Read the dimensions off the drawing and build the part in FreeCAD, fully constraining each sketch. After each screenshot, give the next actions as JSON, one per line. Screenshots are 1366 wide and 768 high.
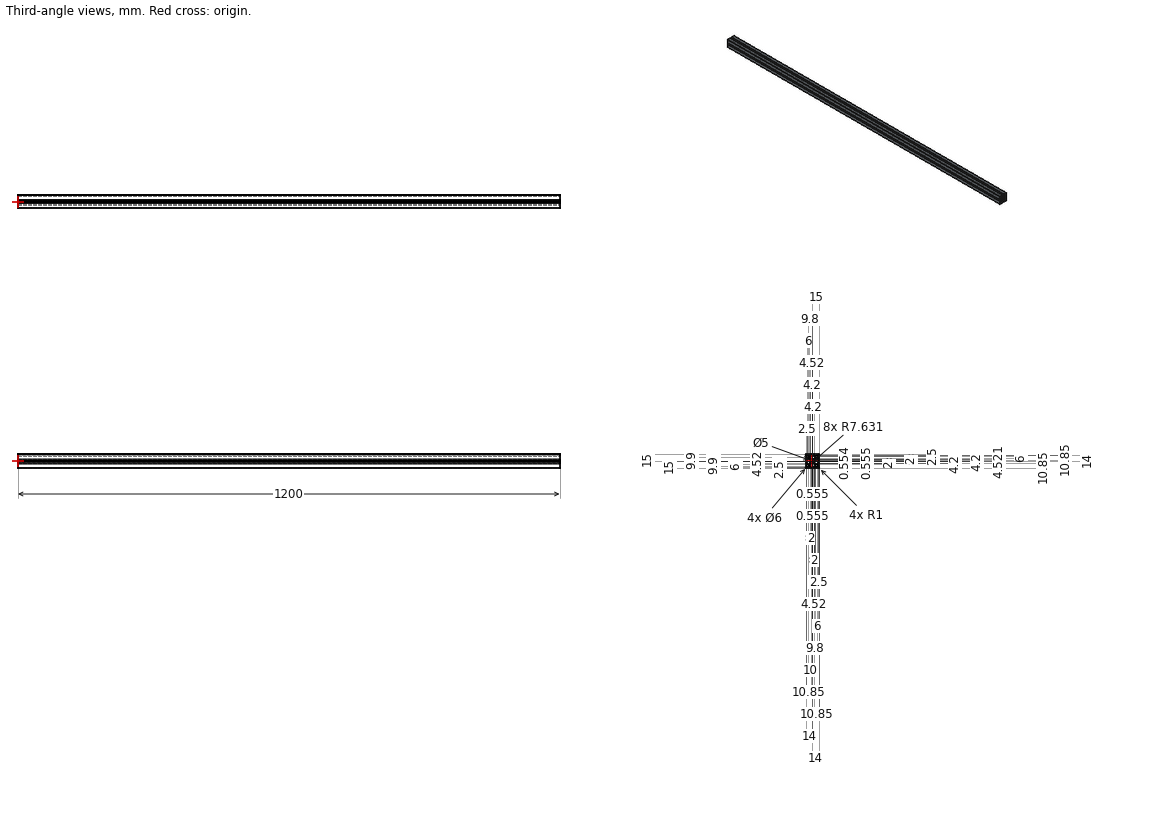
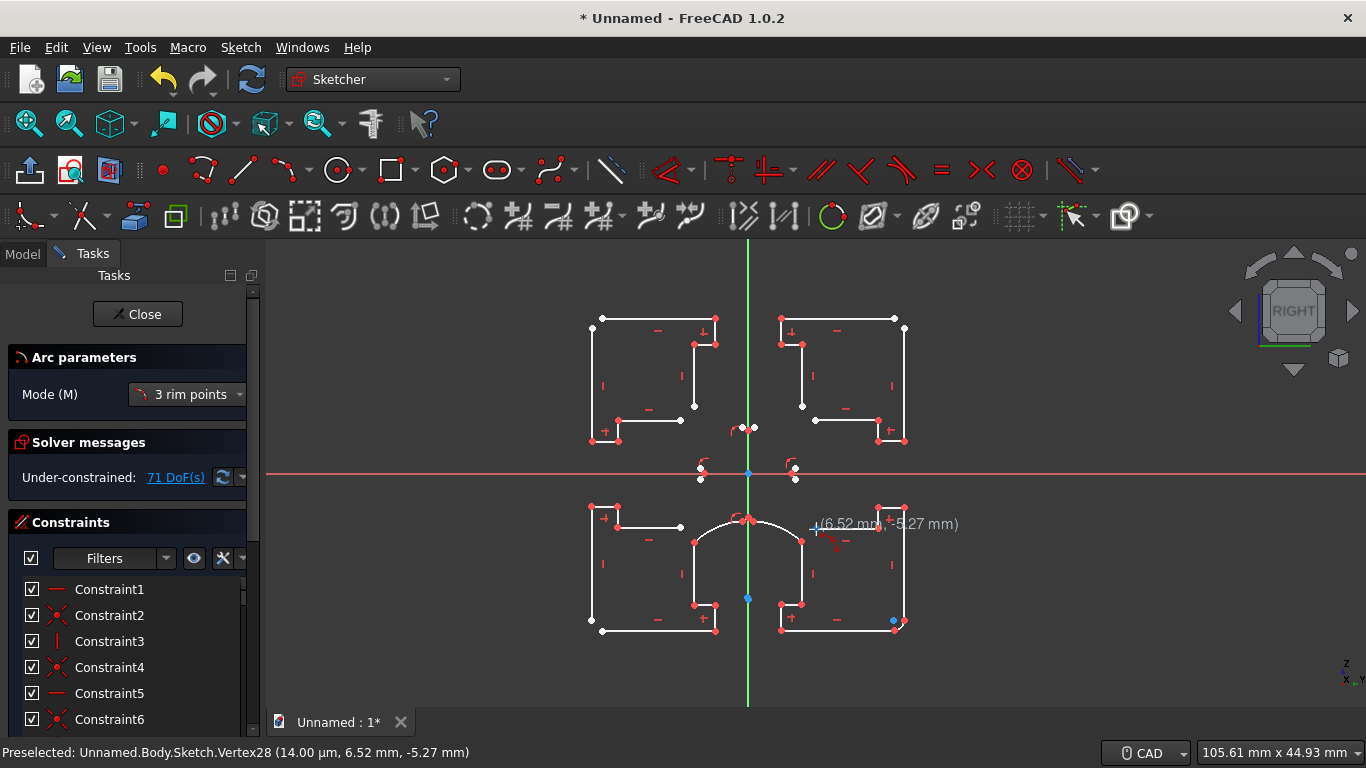
{"action": "scroll", "coordinate": [795, 480], "scroll_direction": "up", "scroll_amount": 8}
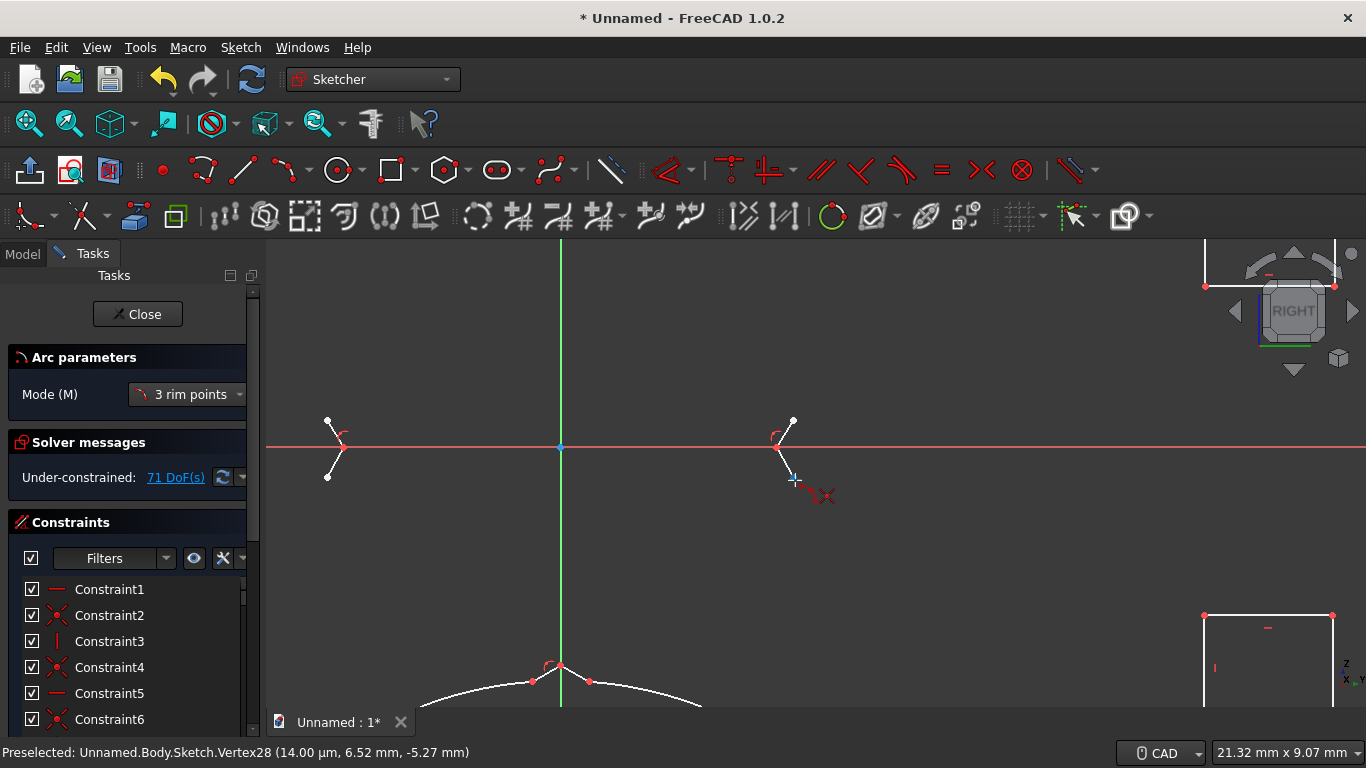
{"action": "left_click", "coordinate": [793, 477]}
{"action": "left_click", "coordinate": [825, 603]}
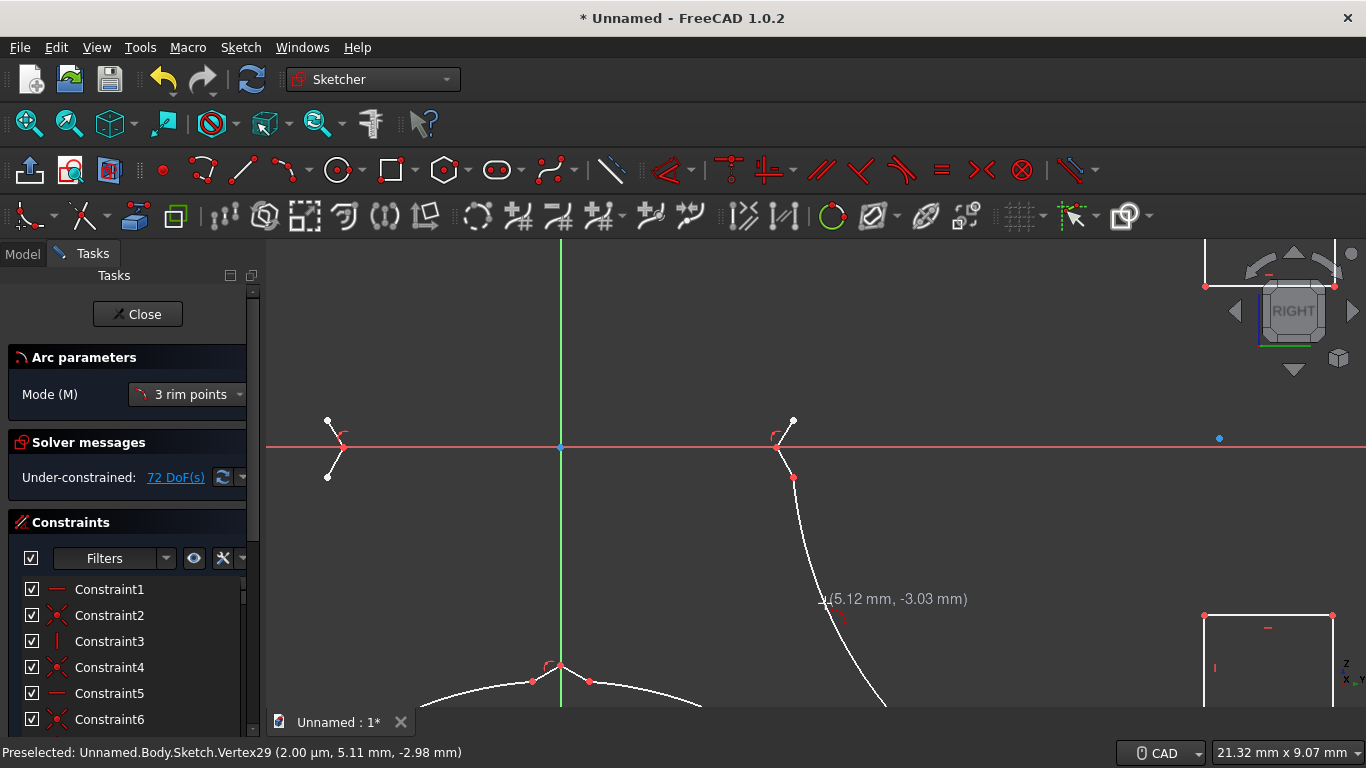
{"action": "left_click", "coordinate": [793, 420]}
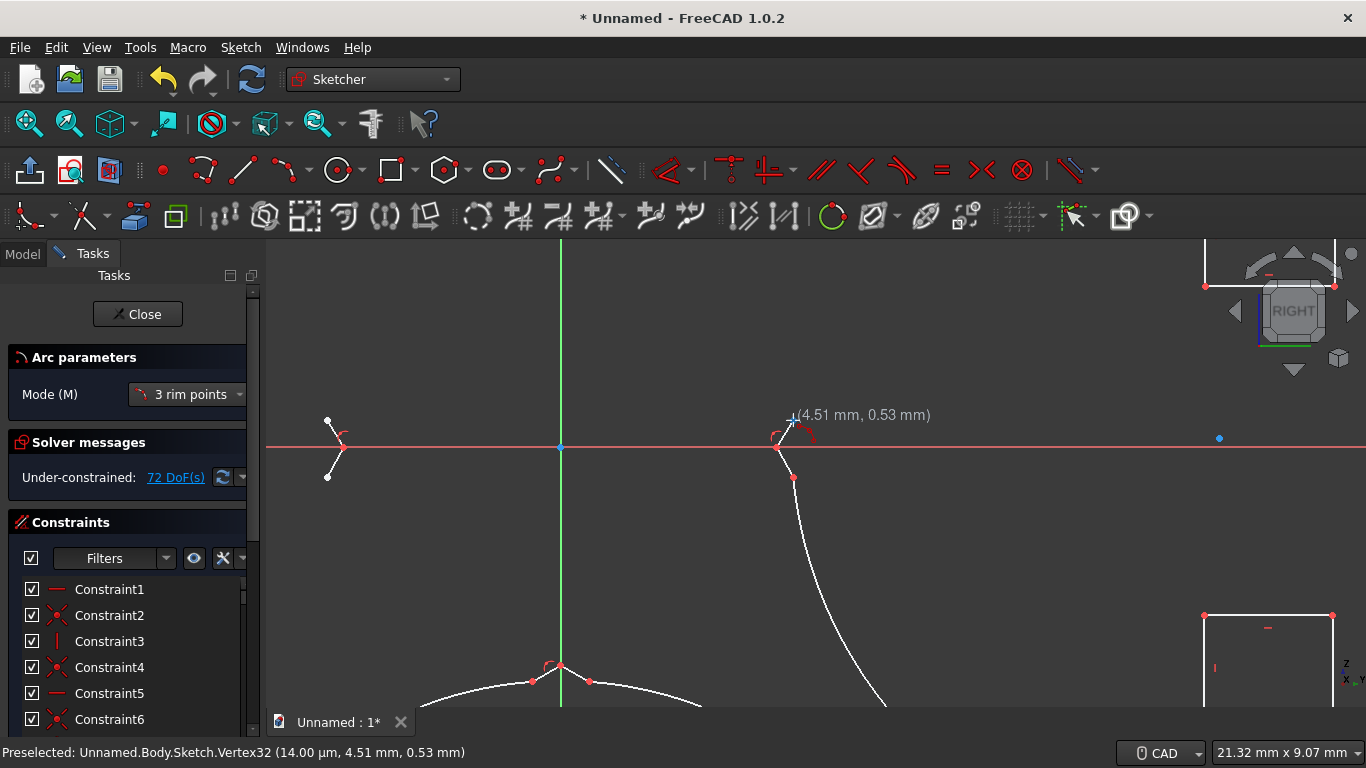
{"action": "scroll", "coordinate": [795, 479], "scroll_direction": "down", "scroll_amount": 8}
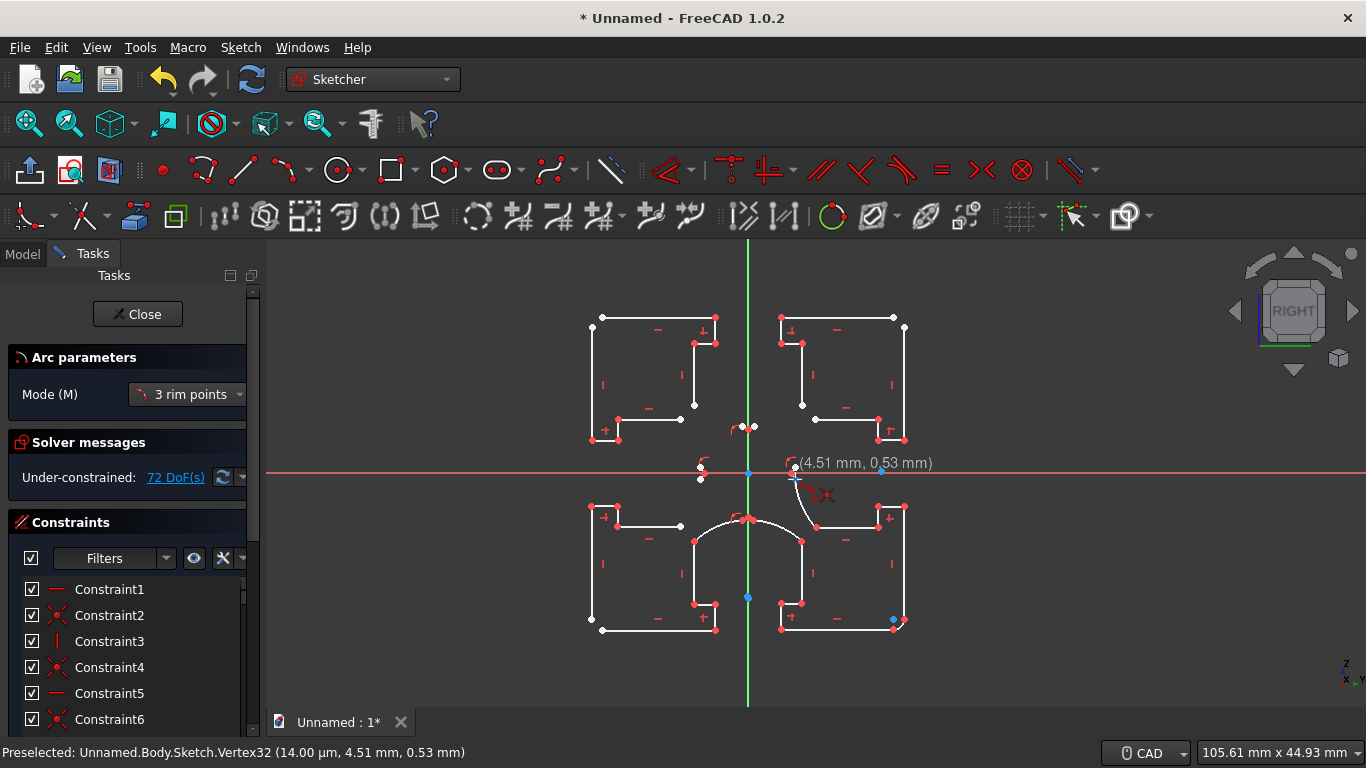
{"action": "left_click", "coordinate": [816, 420]}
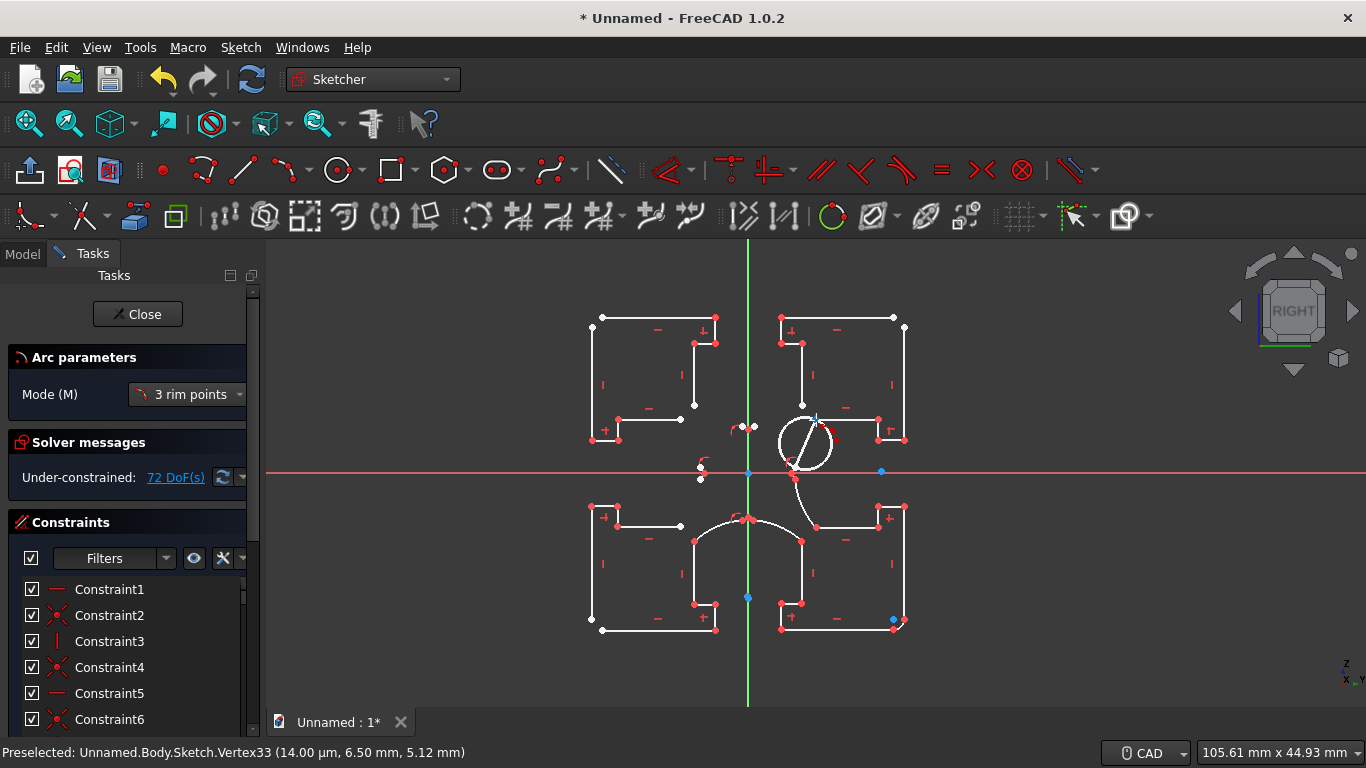
{"action": "scroll", "coordinate": [801, 442], "scroll_direction": "up", "scroll_amount": 7}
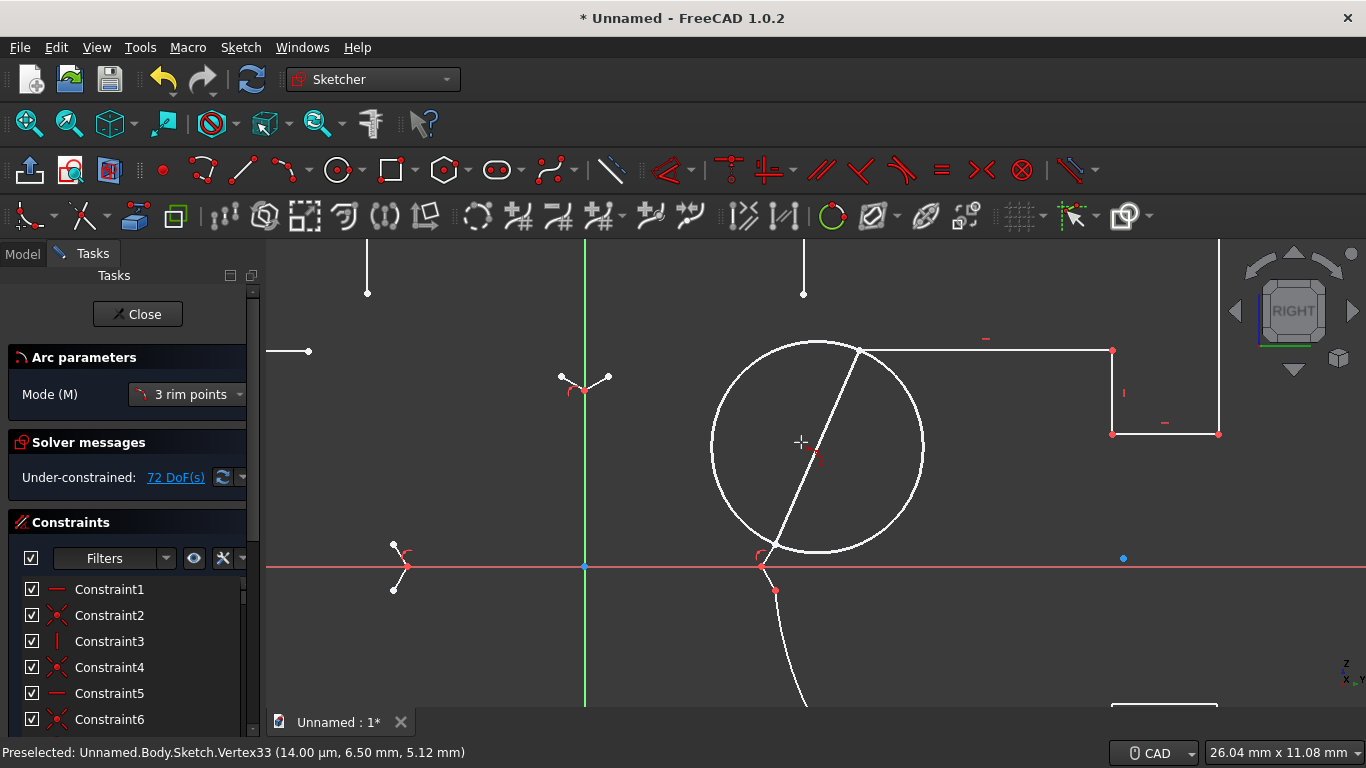
{"action": "left_click", "coordinate": [801, 439]}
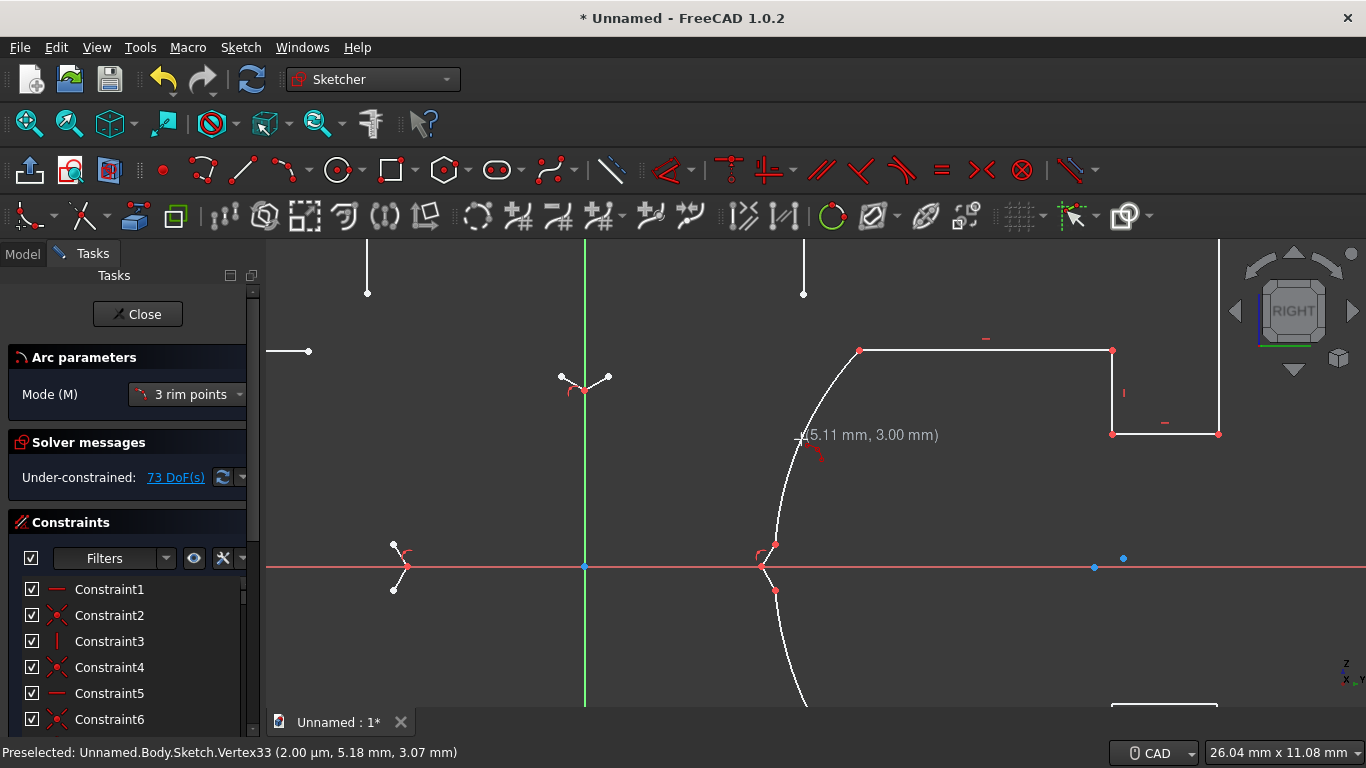
{"action": "scroll", "coordinate": [801, 442], "scroll_direction": "down", "scroll_amount": 7}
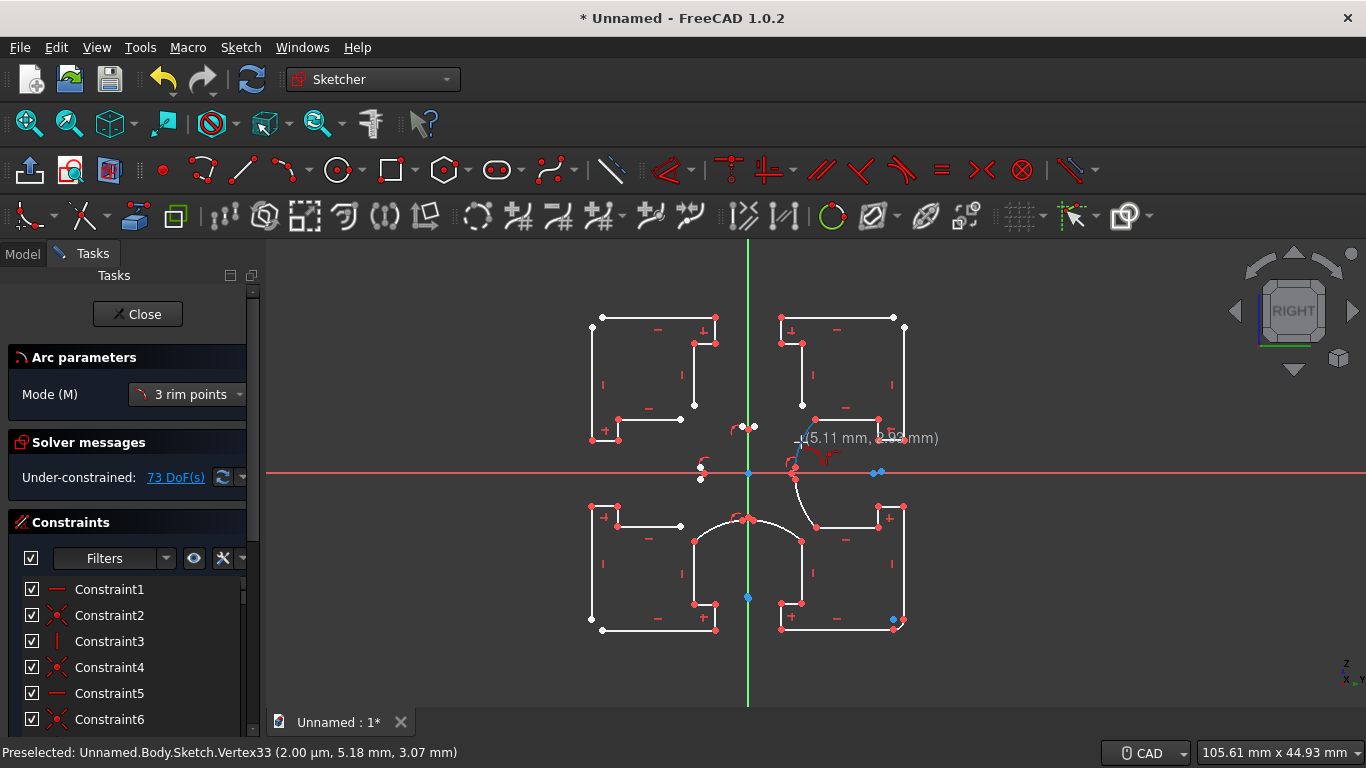
{"action": "left_click", "coordinate": [904, 328]}
{"action": "left_click", "coordinate": [894, 318]}